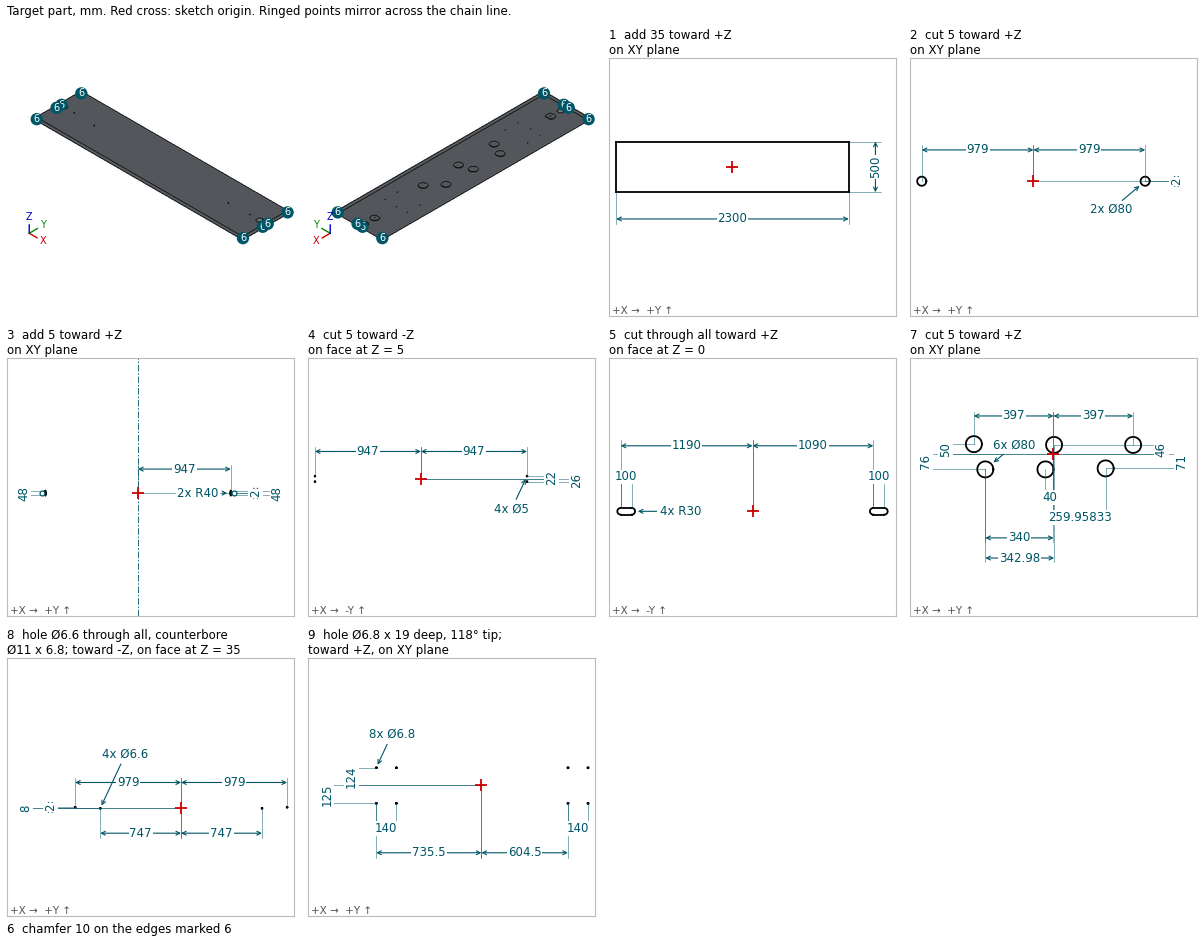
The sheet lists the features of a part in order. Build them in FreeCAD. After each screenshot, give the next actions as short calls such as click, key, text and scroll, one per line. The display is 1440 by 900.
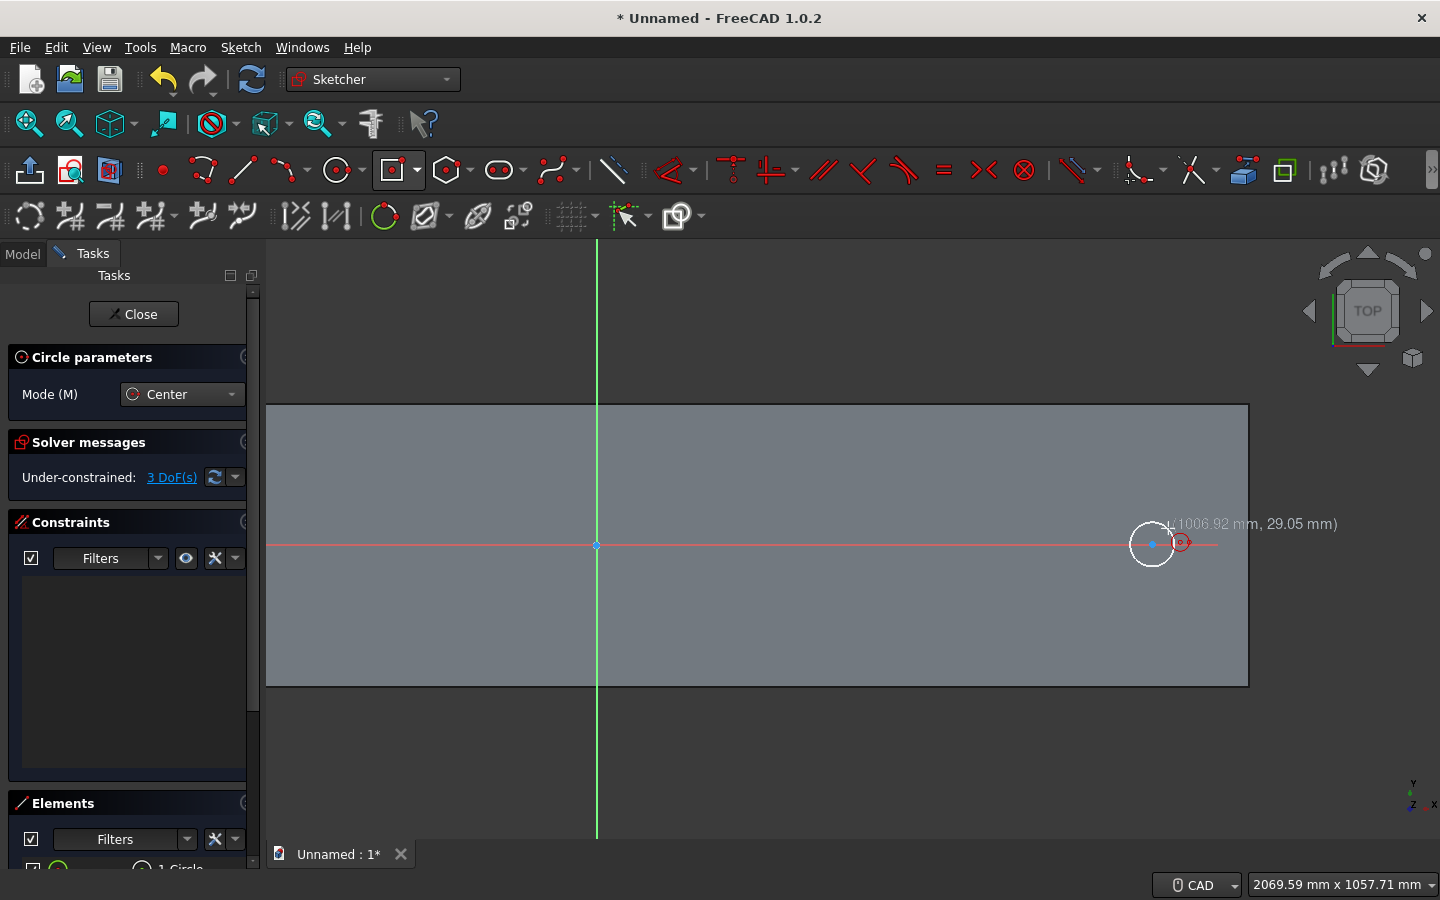
scroll(1013, 532, down, 3)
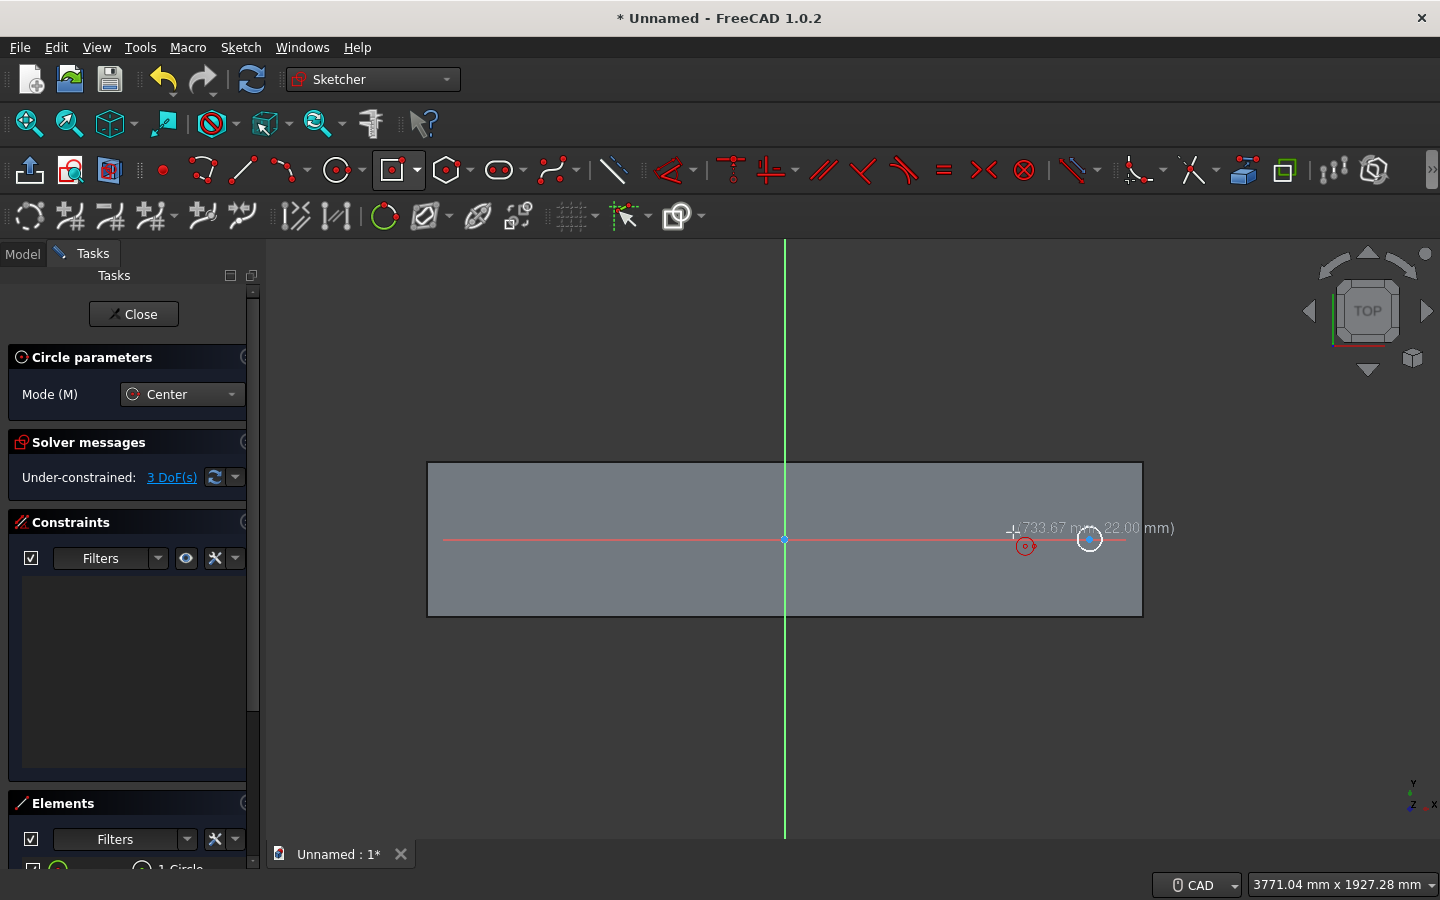
scroll(480, 539, up, 17)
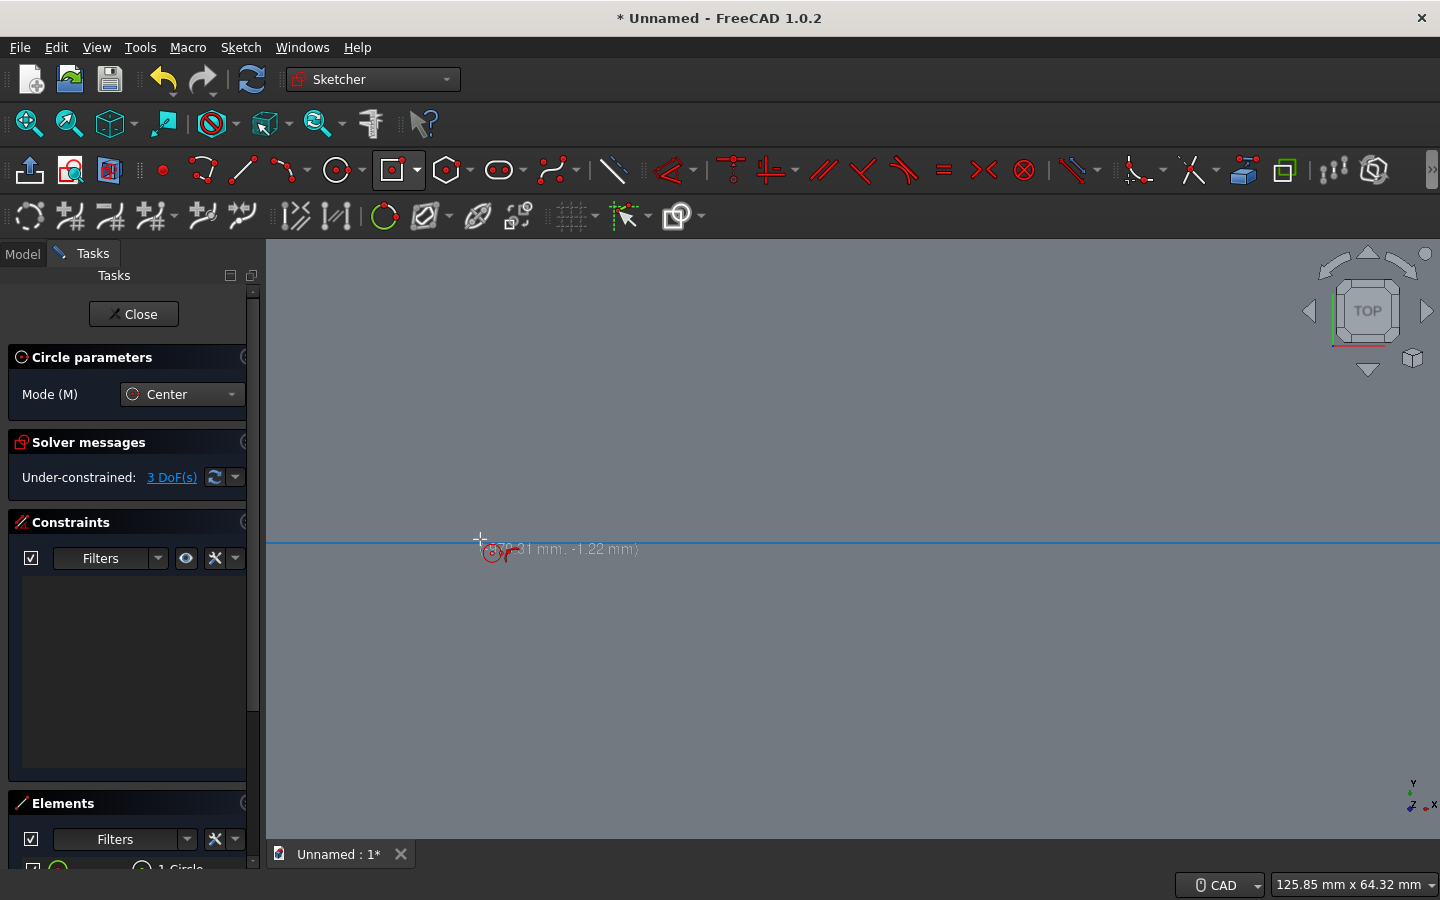
click(478, 524)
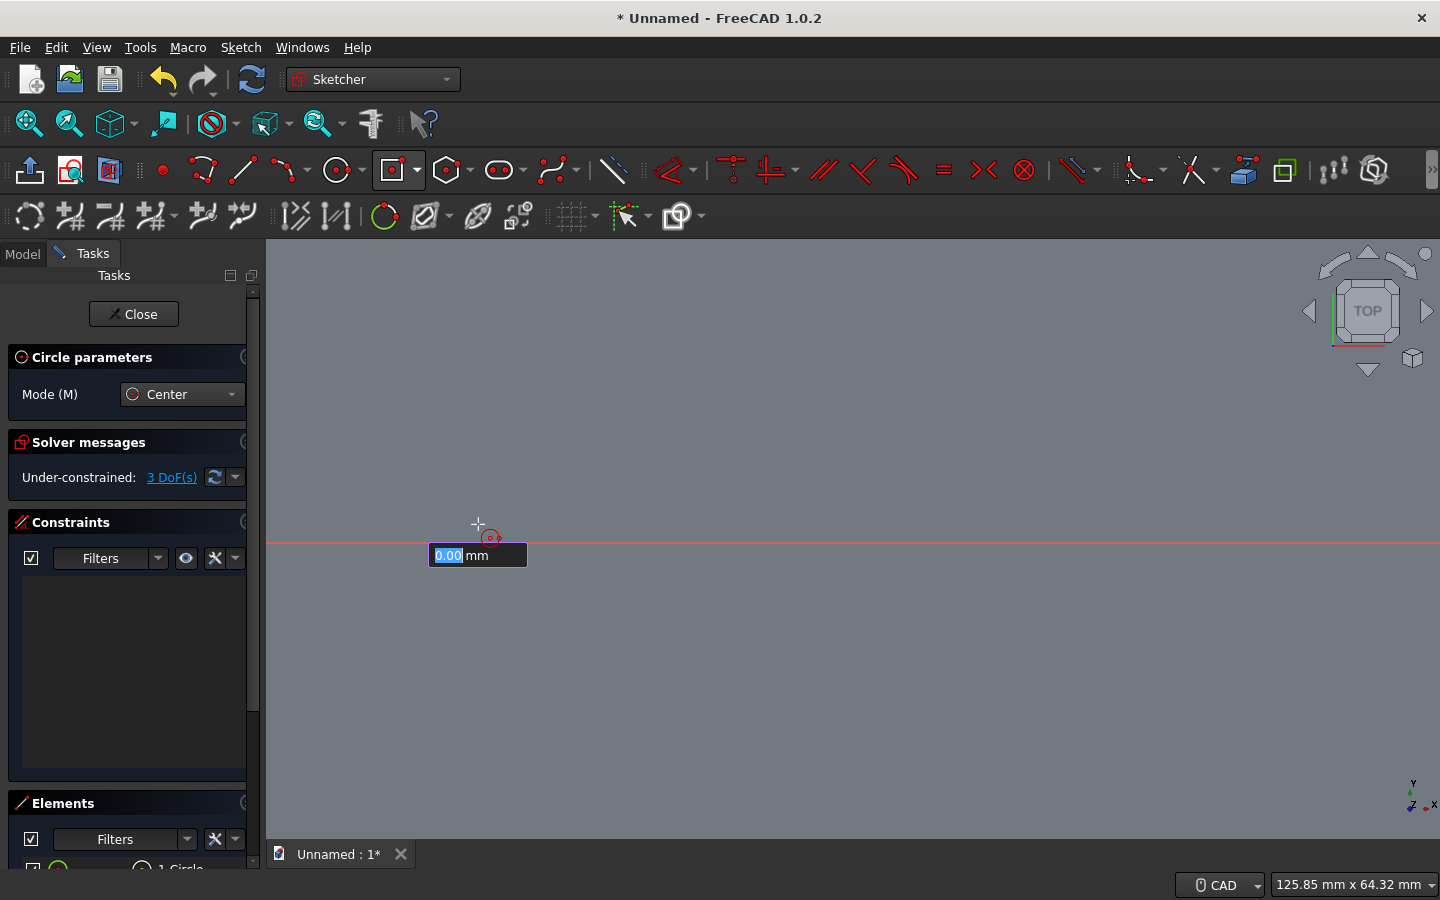
scroll(409, 540, down, 16)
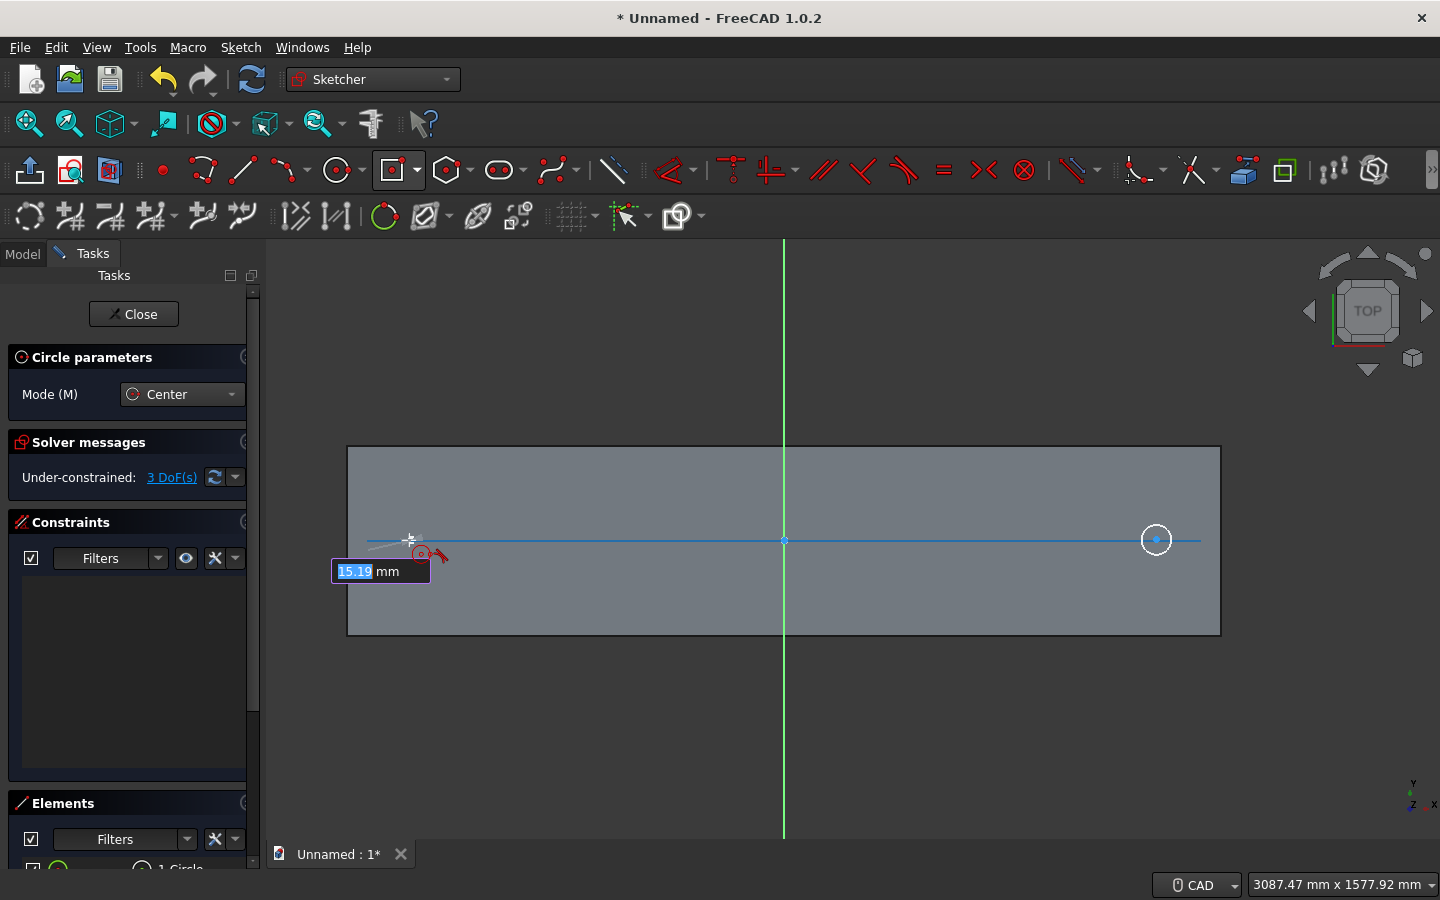
scroll(423, 529, up, 2)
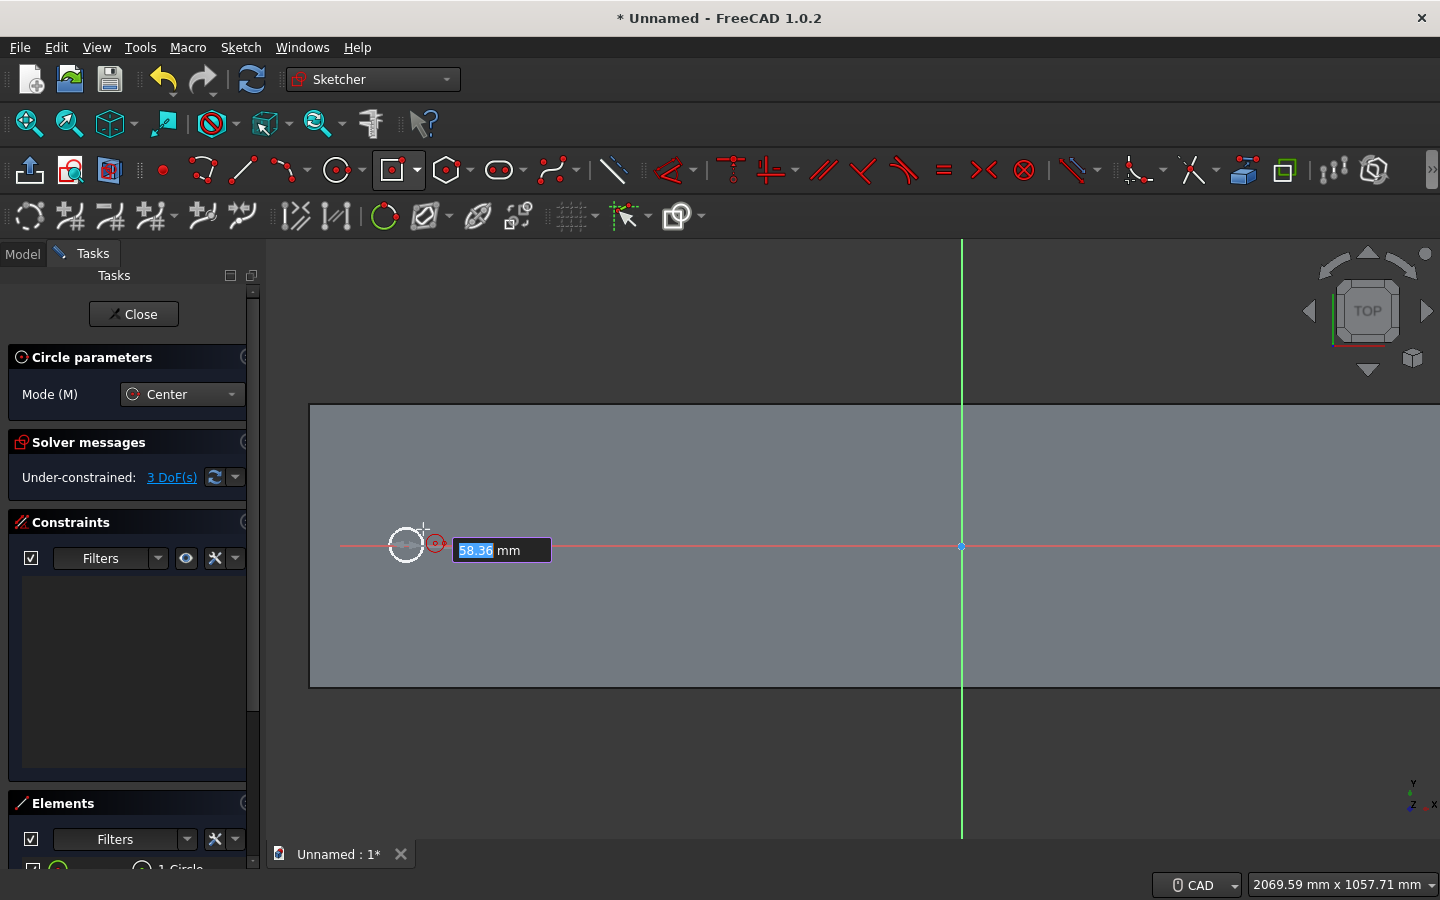
click(422, 529)
key(Escape)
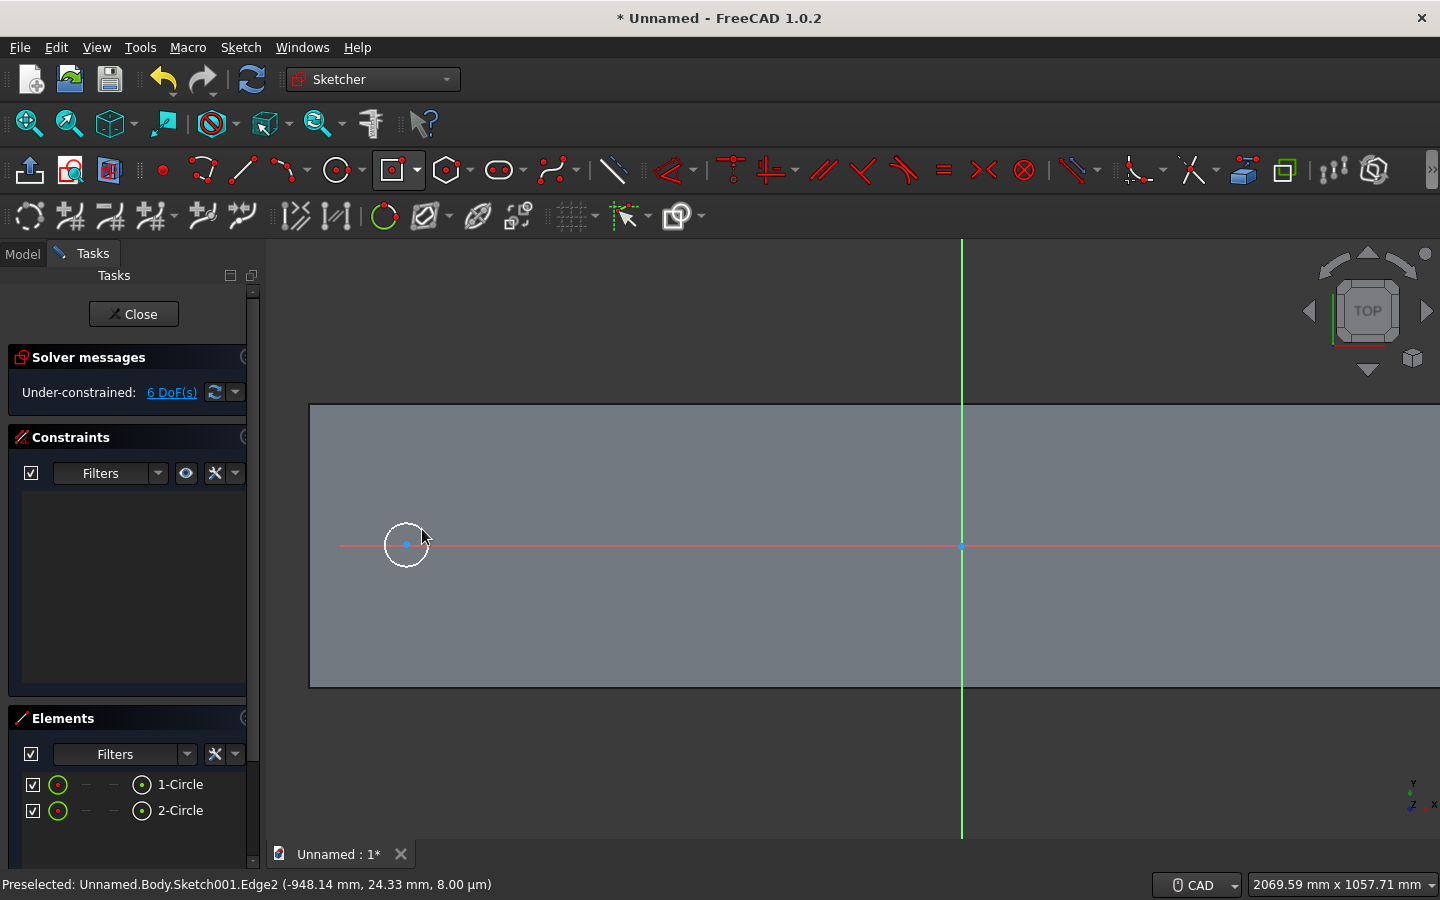
scroll(569, 532, down, 3)